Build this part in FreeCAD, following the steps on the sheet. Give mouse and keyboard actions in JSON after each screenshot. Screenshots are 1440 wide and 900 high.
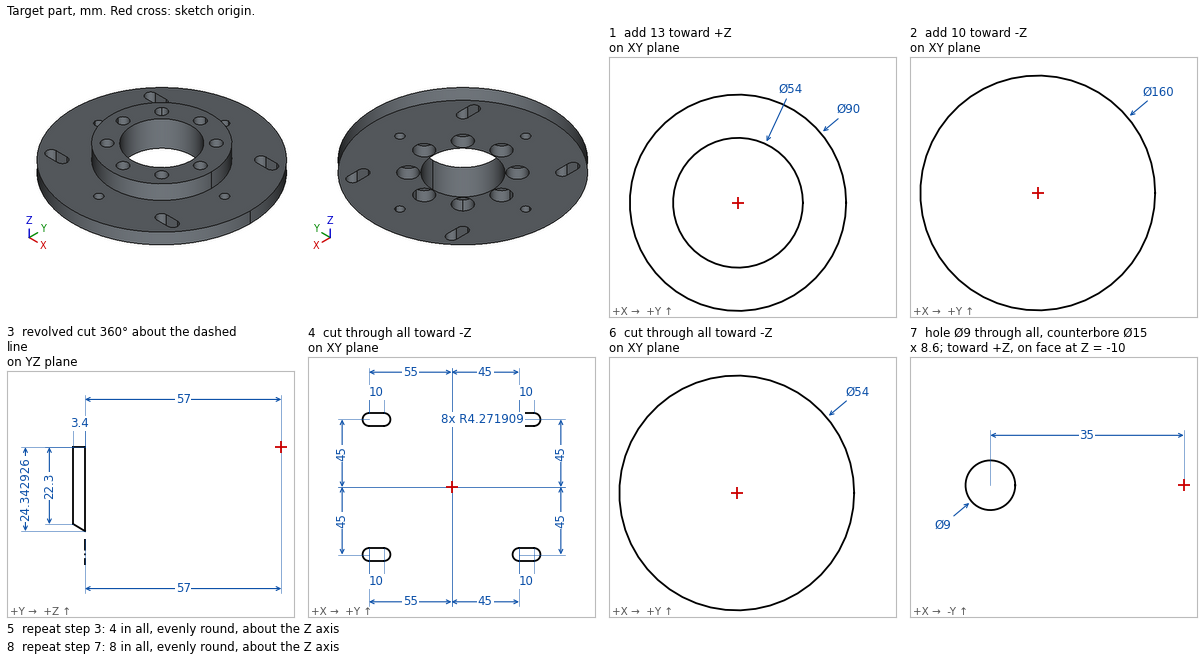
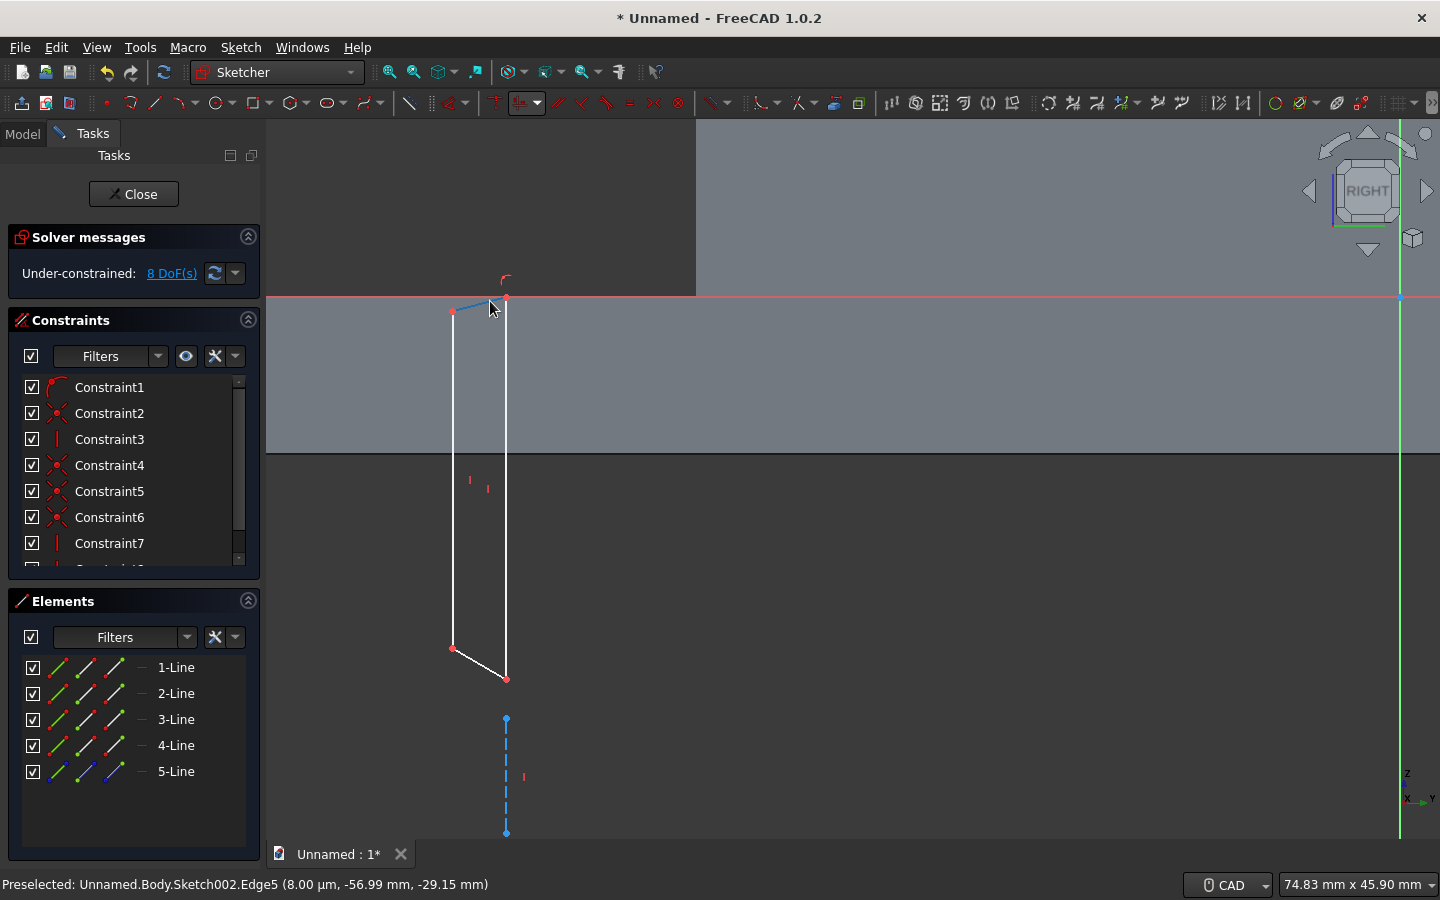
{"action": "left_click", "coordinate": [490, 301]}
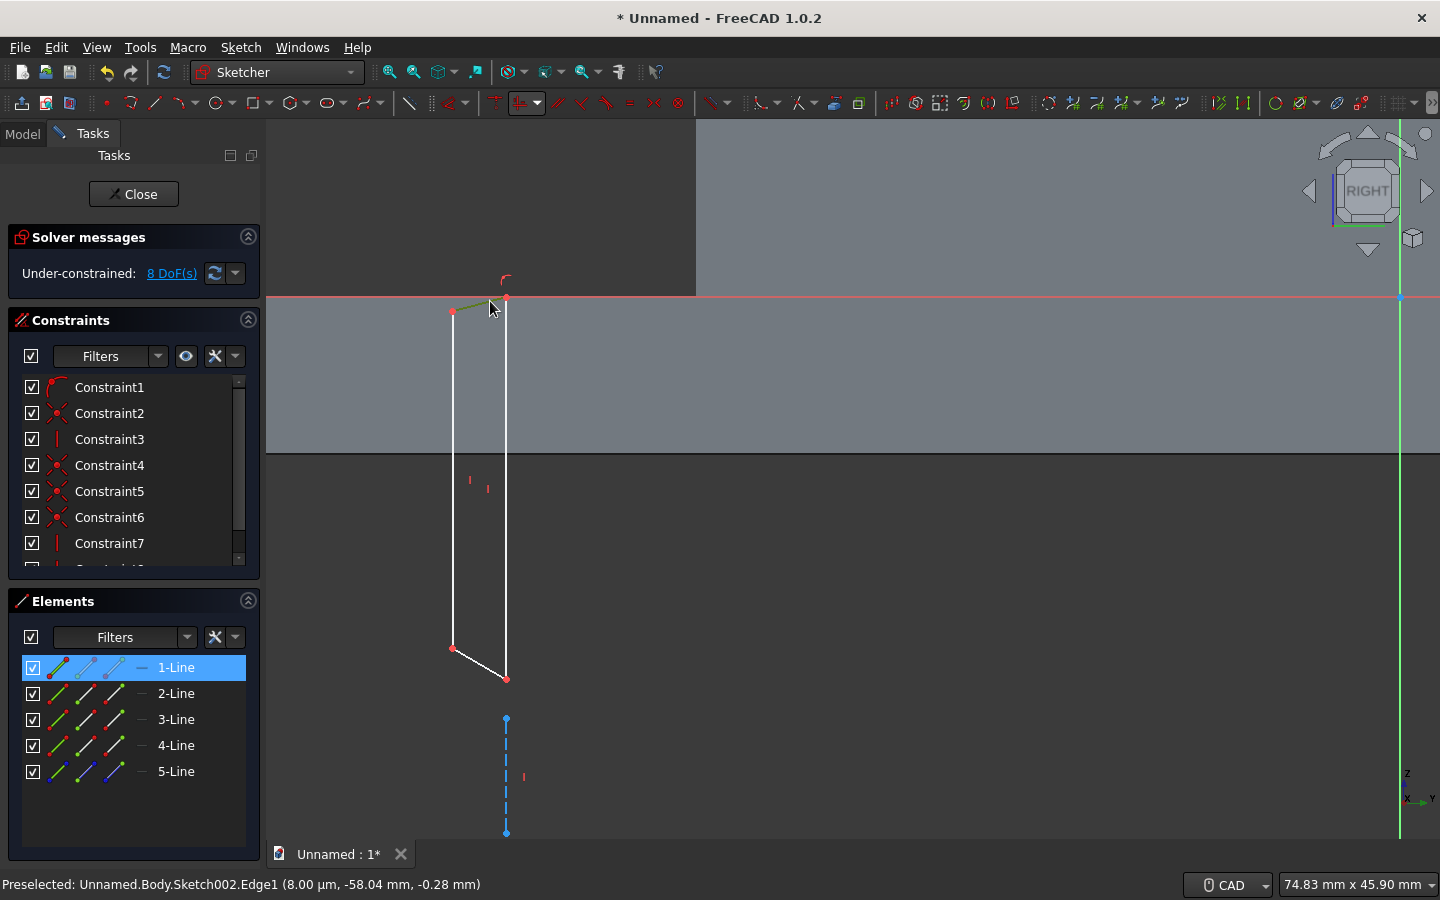
{"action": "key", "text": "h"}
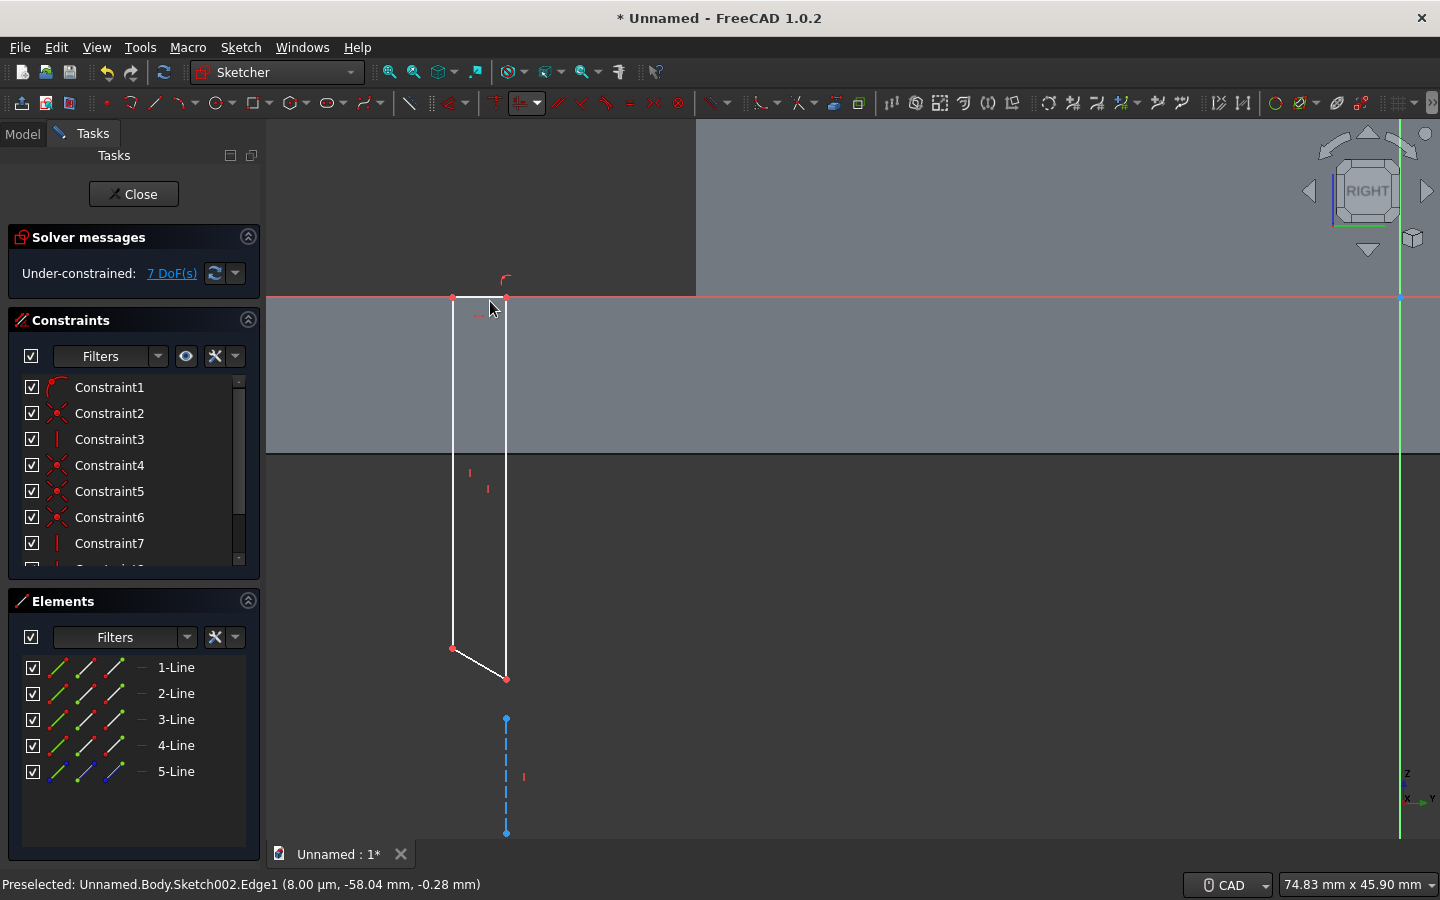
{"action": "key", "text": "d"}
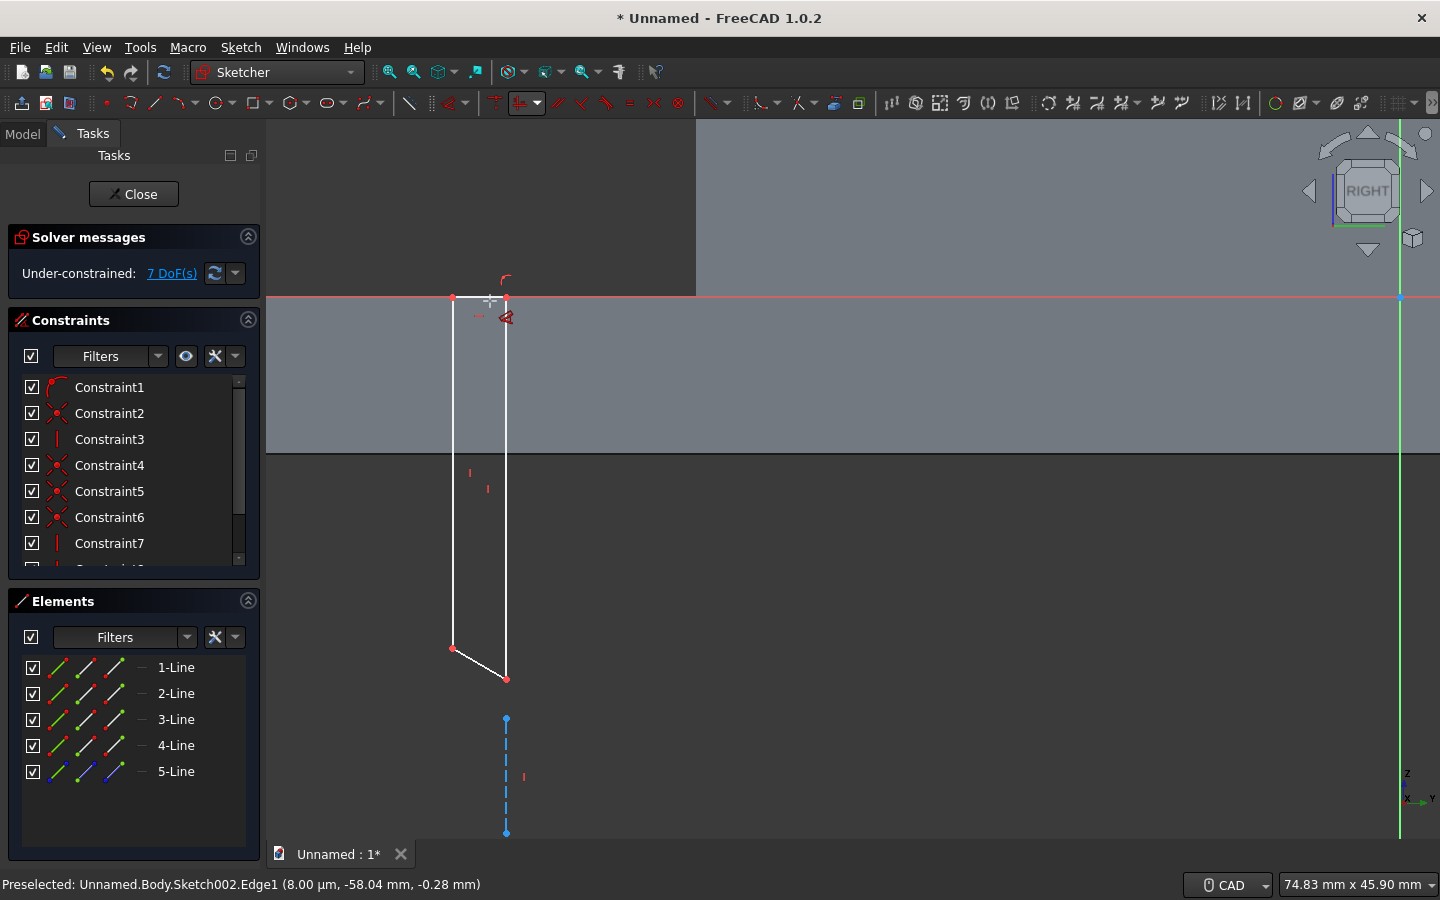
{"action": "left_click", "coordinate": [490, 297]}
{"action": "left_click", "coordinate": [479, 263]}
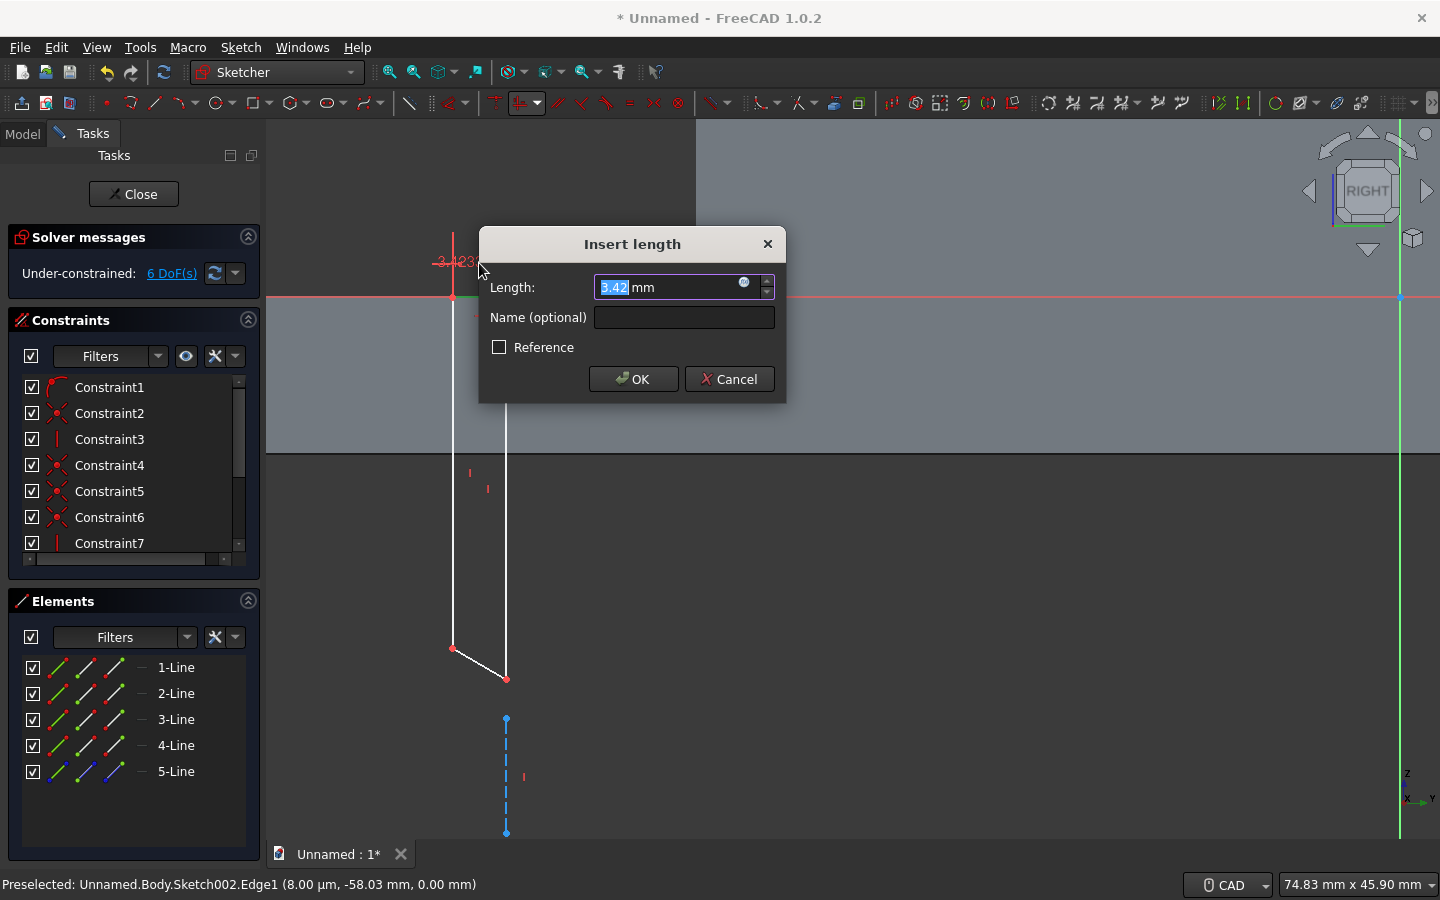
{"action": "type", "text": "3.4"}
{"action": "key", "text": "Return"}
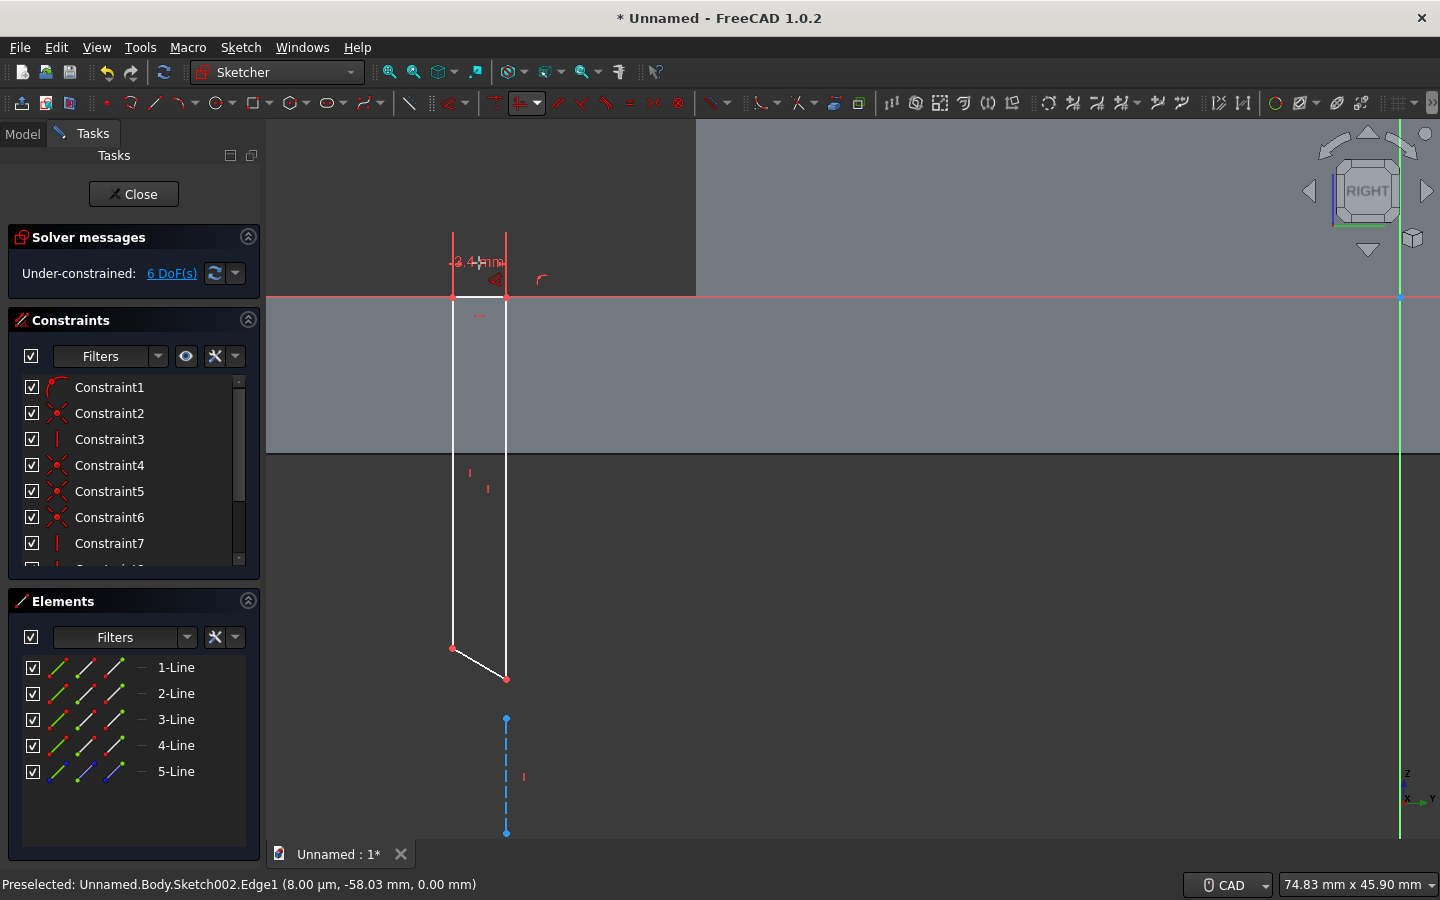
{"action": "left_click", "coordinate": [506, 297]}
{"action": "left_click", "coordinate": [891, 263]}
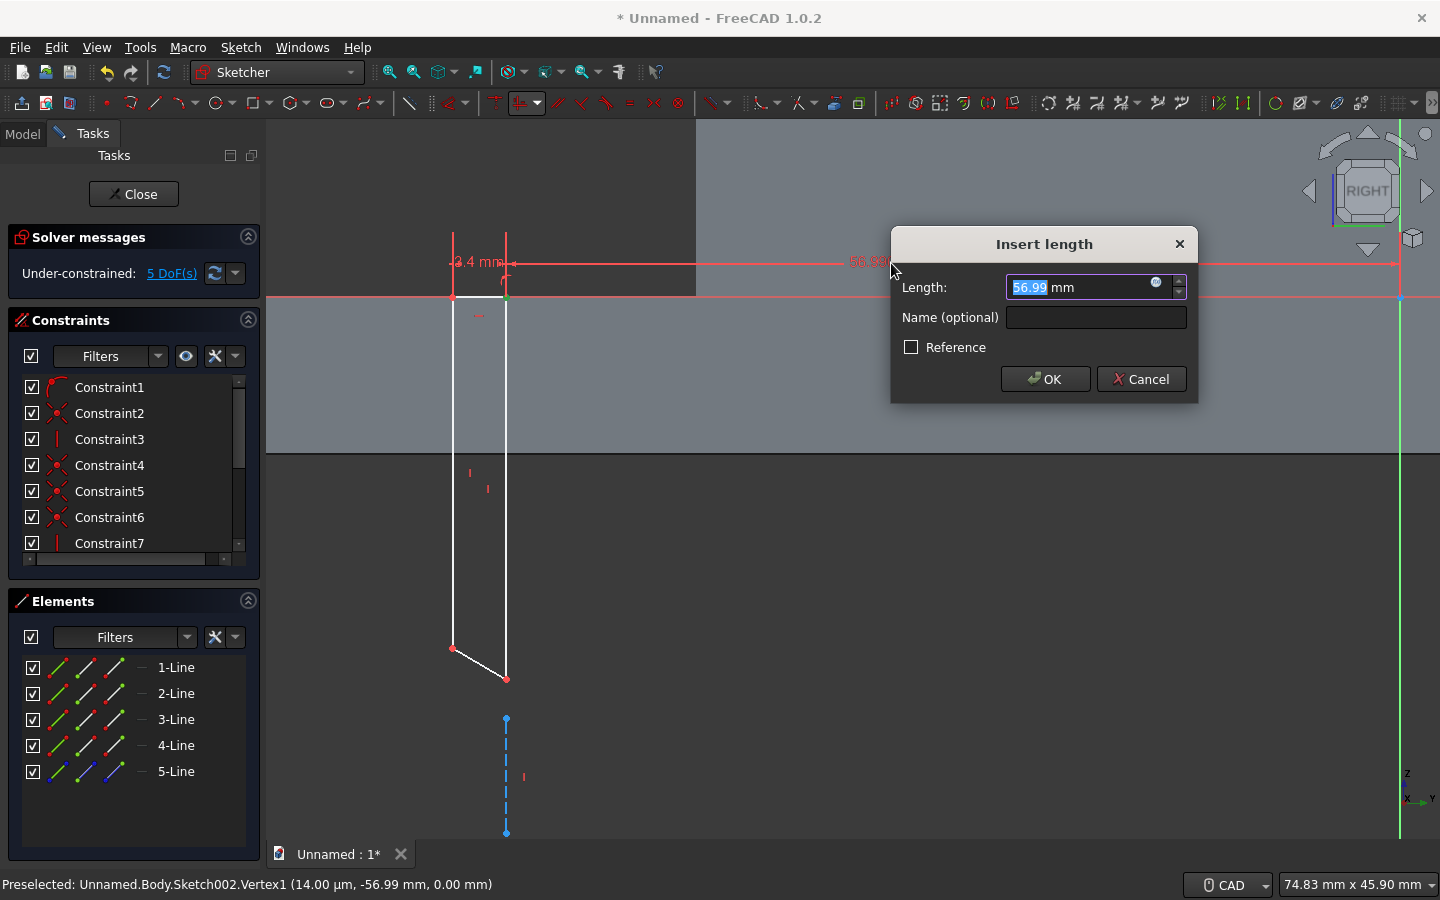
{"action": "type", "text": "57"}
{"action": "key", "text": "Return"}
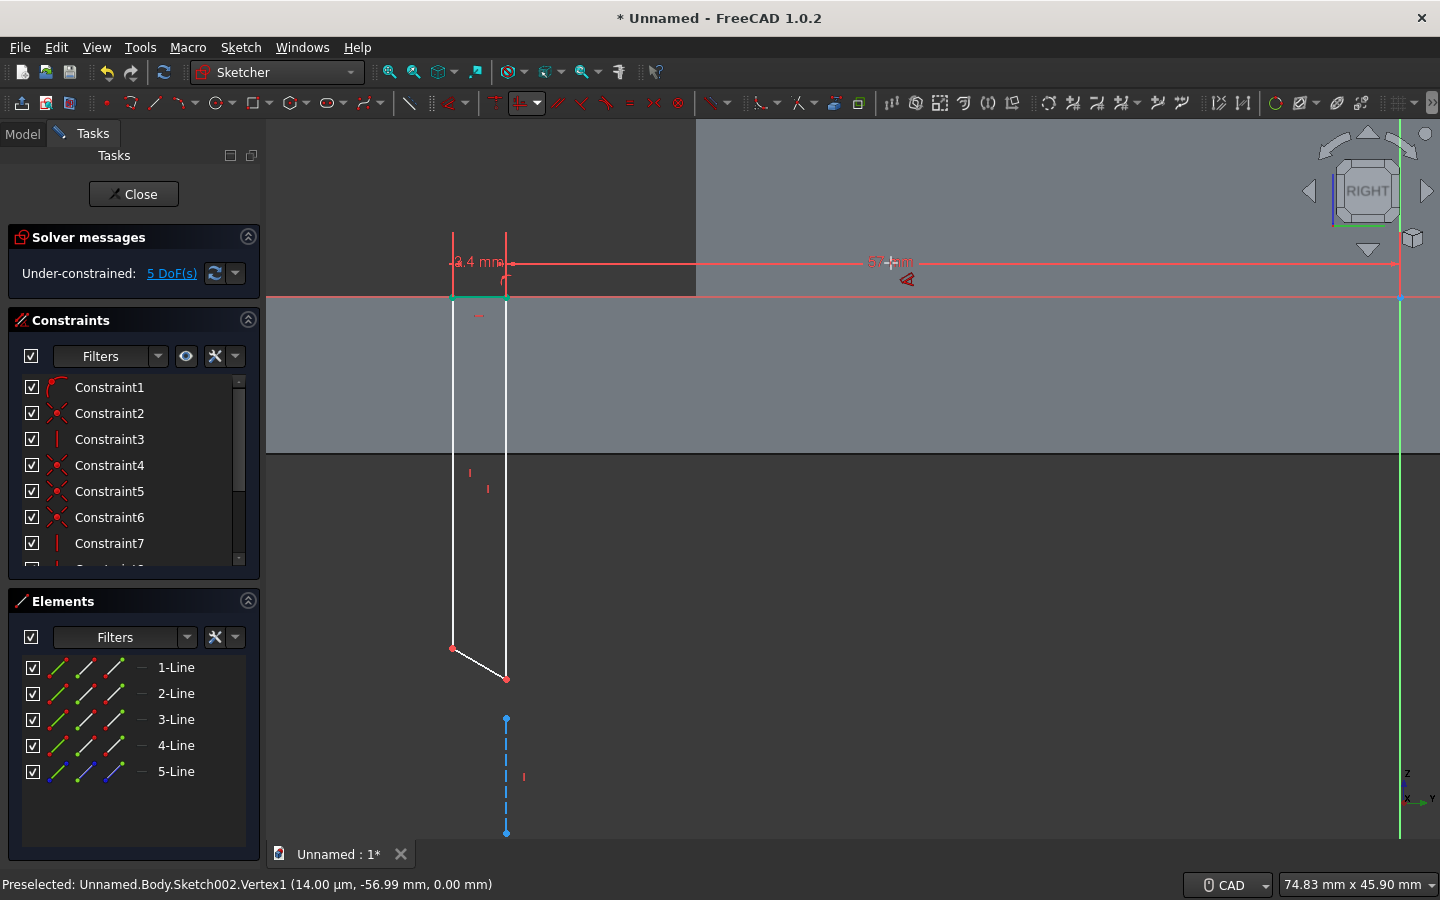
{"action": "left_click", "coordinate": [506, 719]}
{"action": "left_click", "coordinate": [714, 263]}